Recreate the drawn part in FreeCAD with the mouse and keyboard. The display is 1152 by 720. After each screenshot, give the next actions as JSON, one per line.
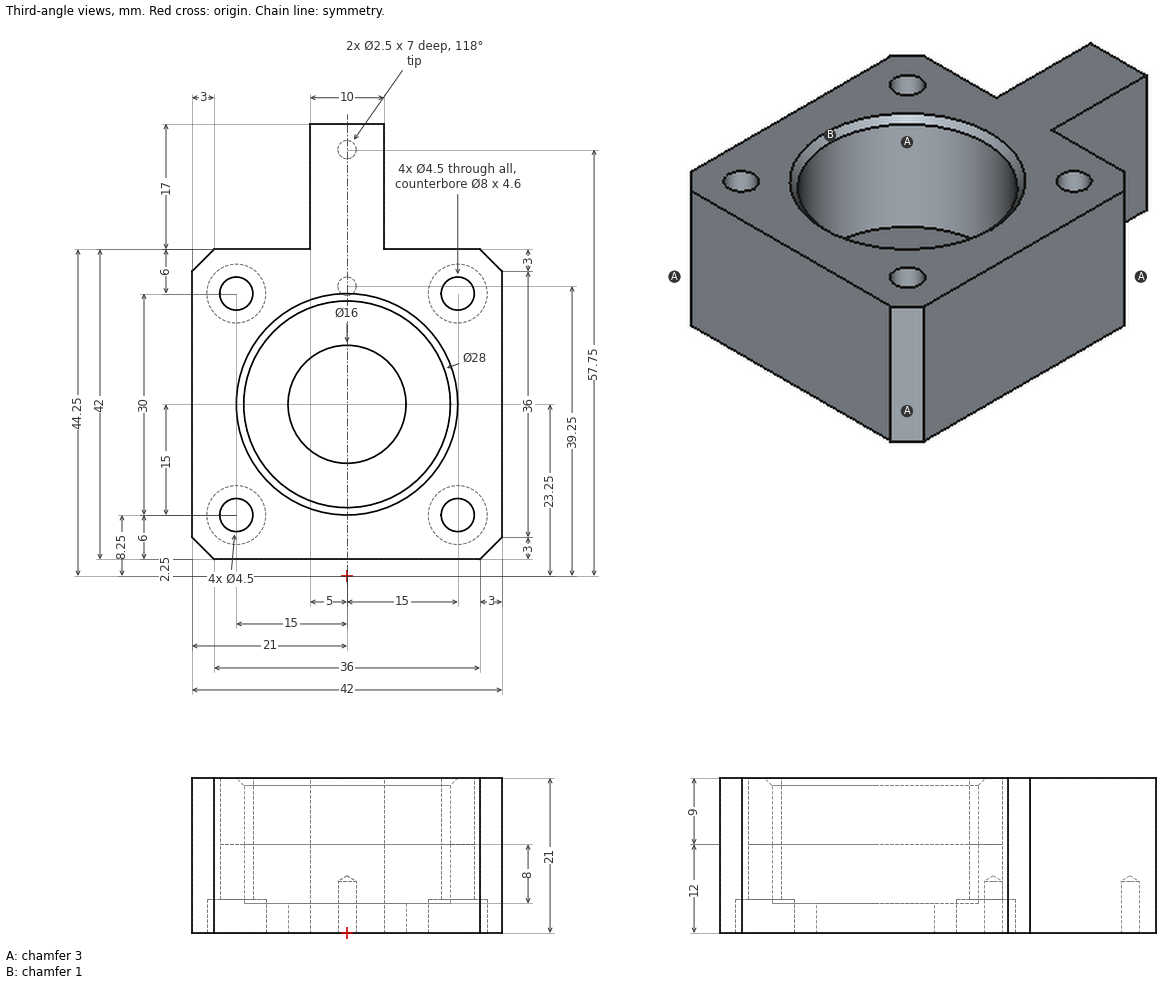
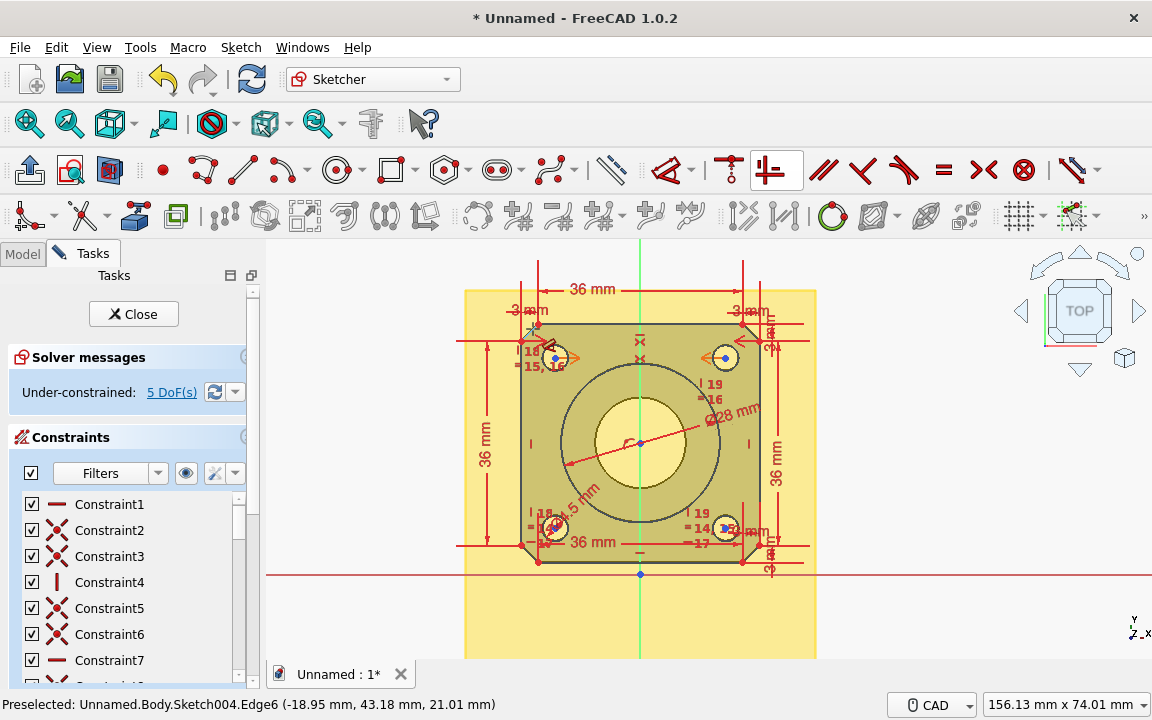
{"action": "left_click", "coordinate": [555, 529]}
{"action": "left_click", "coordinate": [598, 609]}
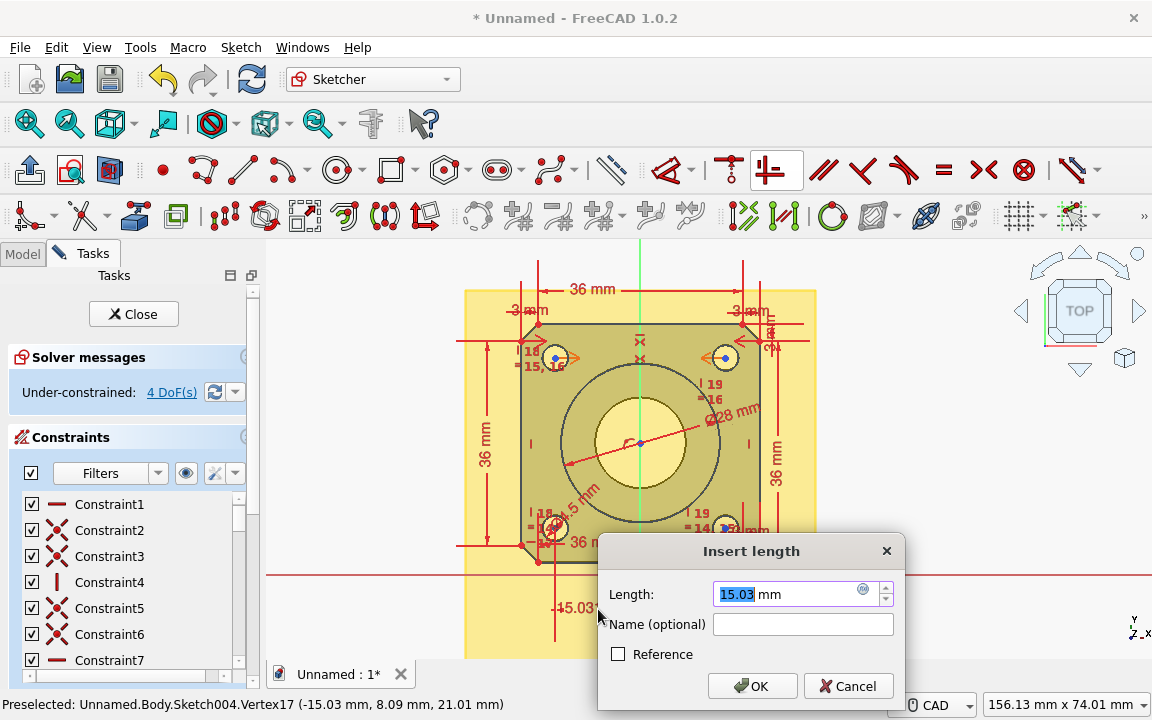
{"action": "type", "text": "15"}
{"action": "key", "text": "Return"}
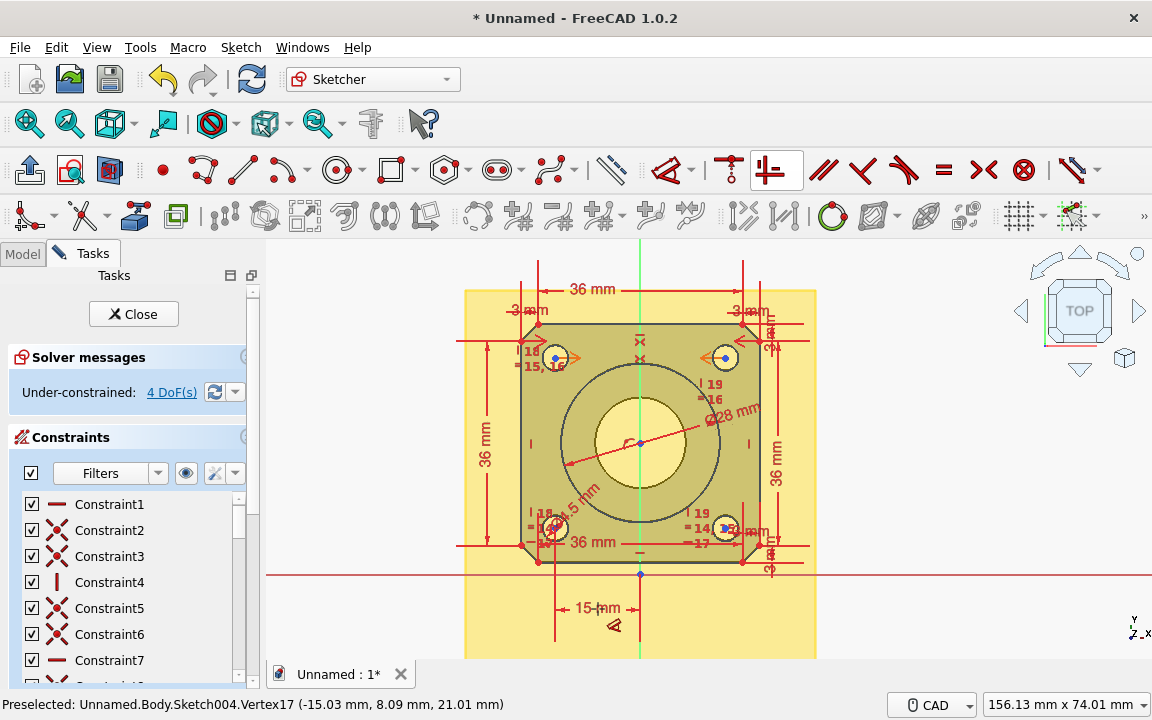
{"action": "left_click", "coordinate": [538, 563]}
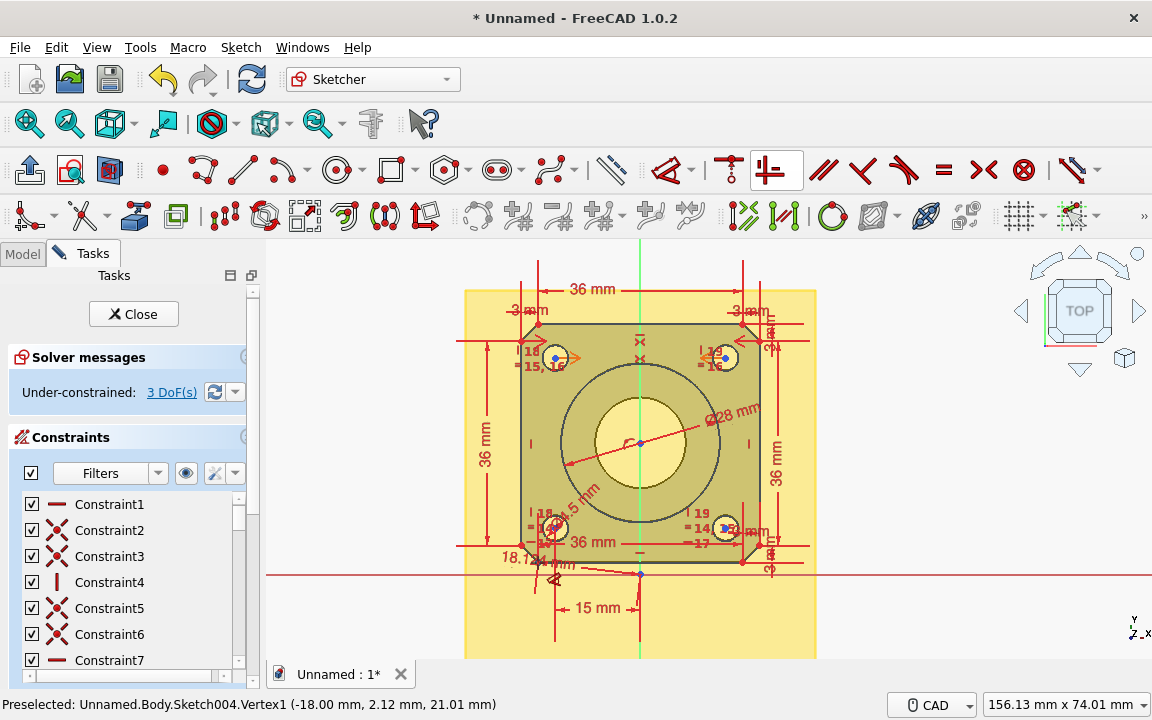
{"action": "left_click", "coordinate": [555, 529]}
{"action": "left_click", "coordinate": [504, 546]}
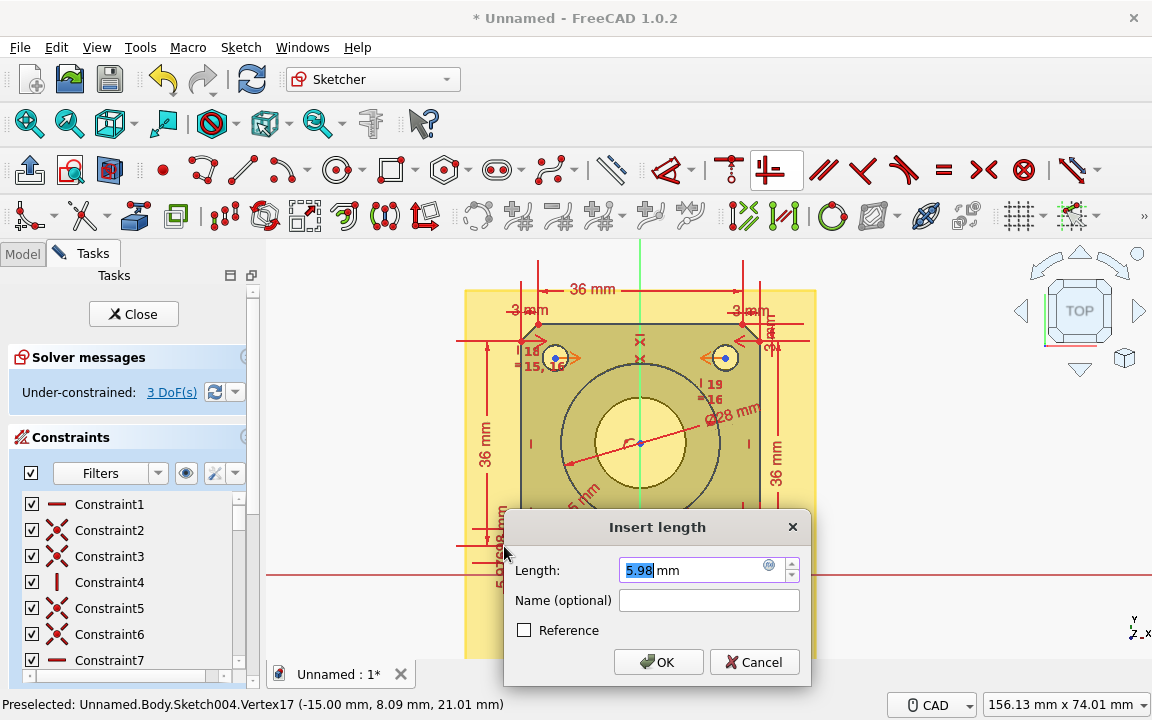
{"action": "type", "text": "6"}
{"action": "key", "text": "Return"}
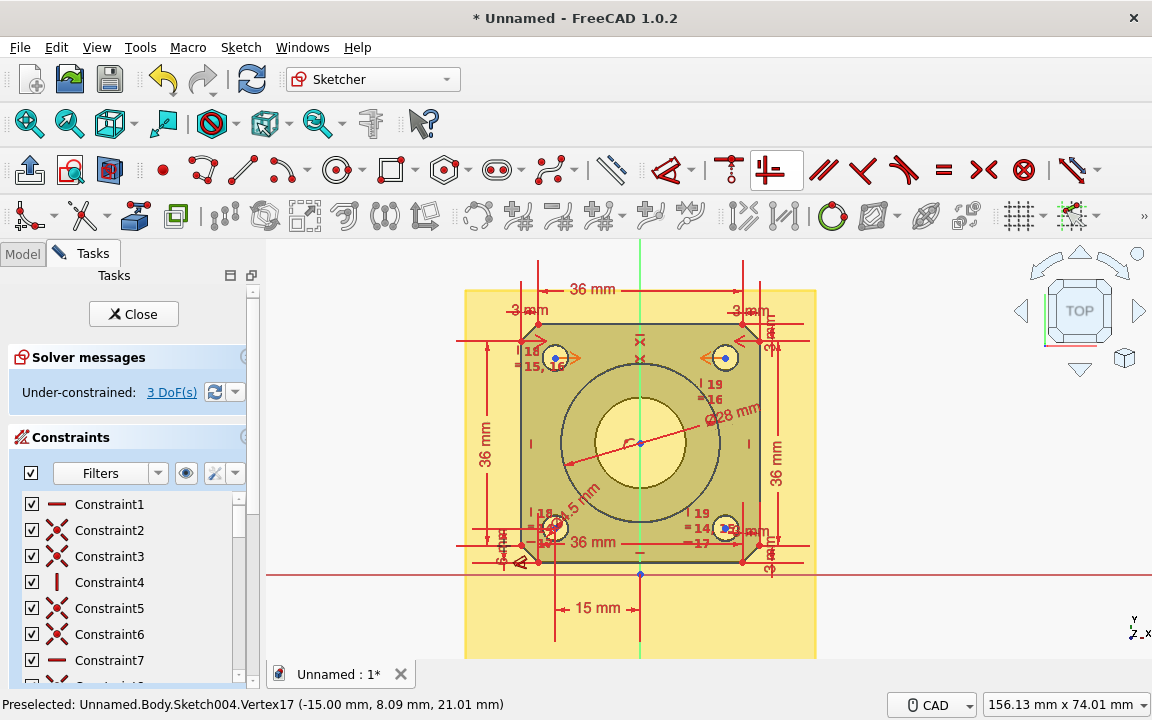
{"action": "left_click", "coordinate": [538, 324]}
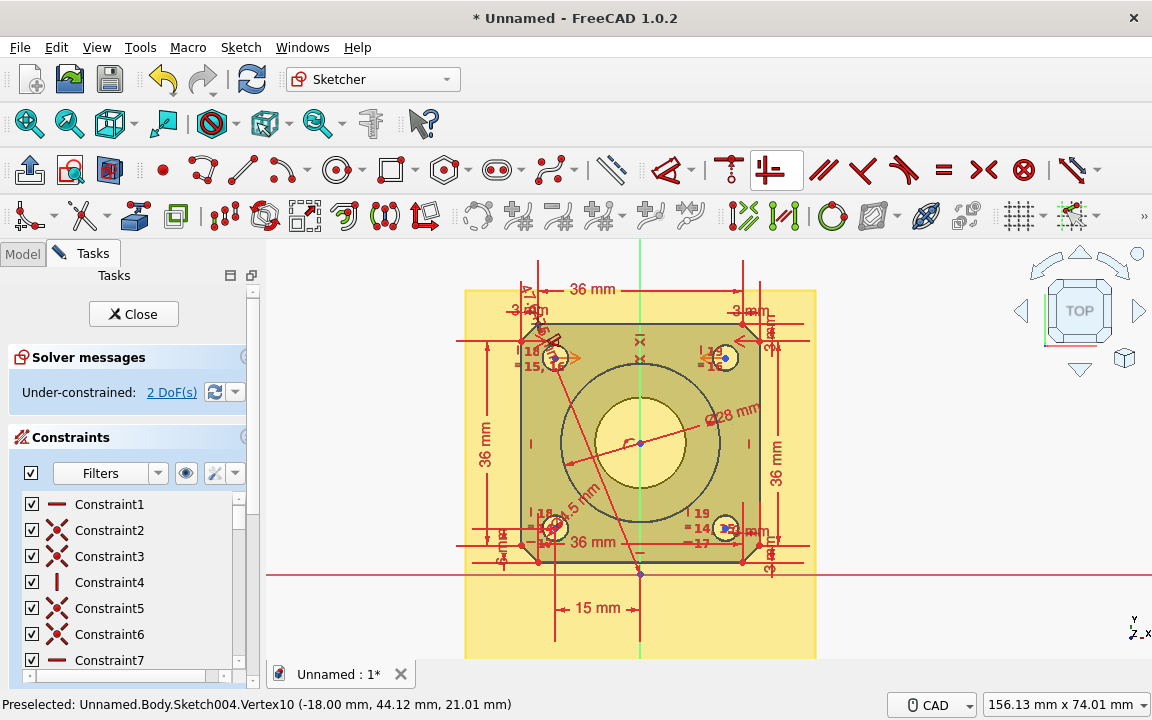
{"action": "left_click", "coordinate": [555, 358]}
{"action": "left_click", "coordinate": [504, 341]}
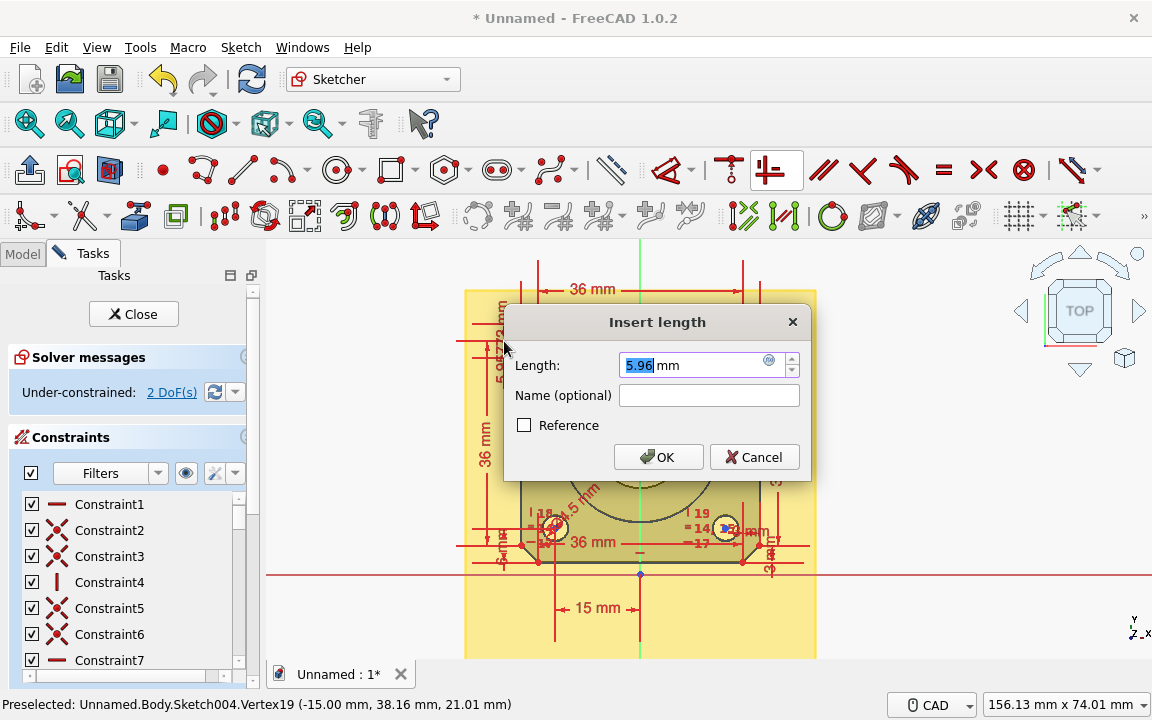
{"action": "type", "text": "6"}
{"action": "key", "text": "Return"}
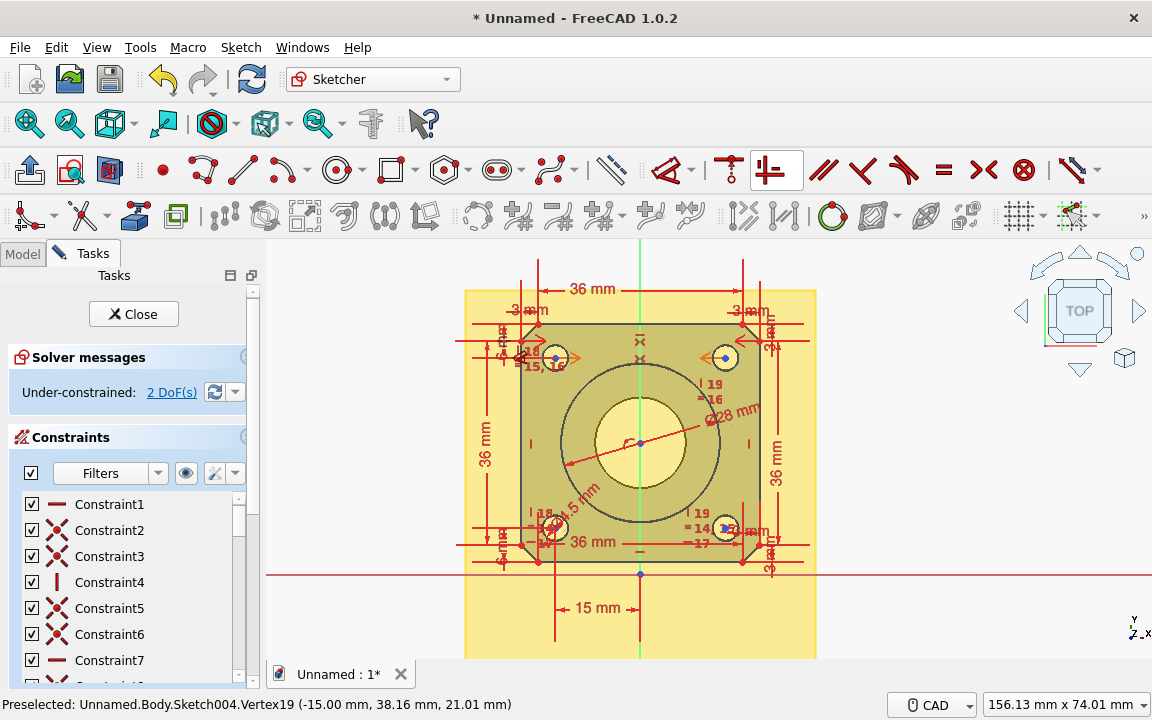
{"action": "left_click", "coordinate": [555, 528]}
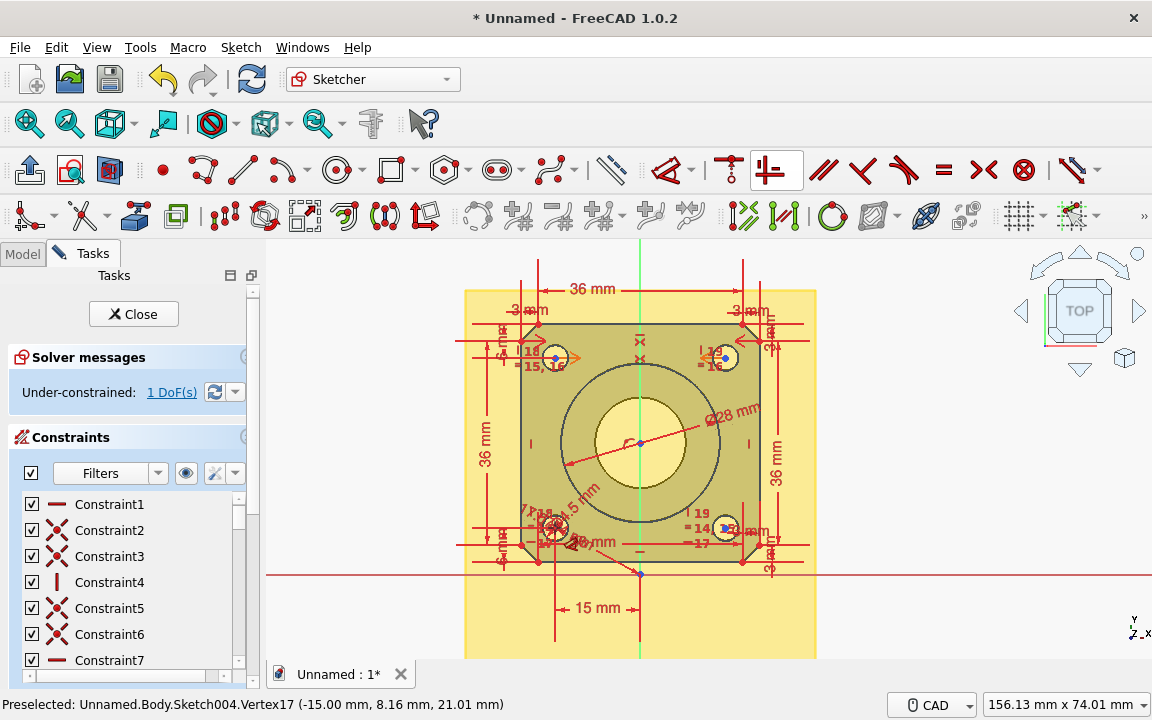
{"action": "left_click", "coordinate": [640, 443]}
{"action": "left_click", "coordinate": [674, 486]}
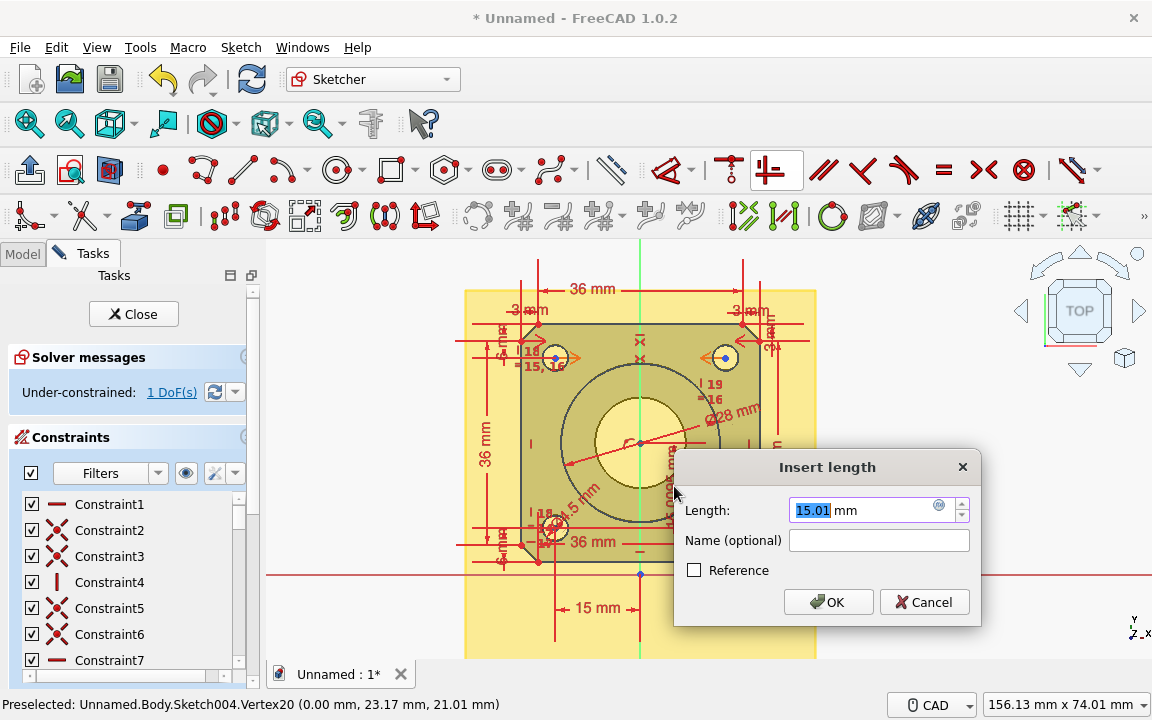
{"action": "type", "text": "15"}
{"action": "key", "text": "Return"}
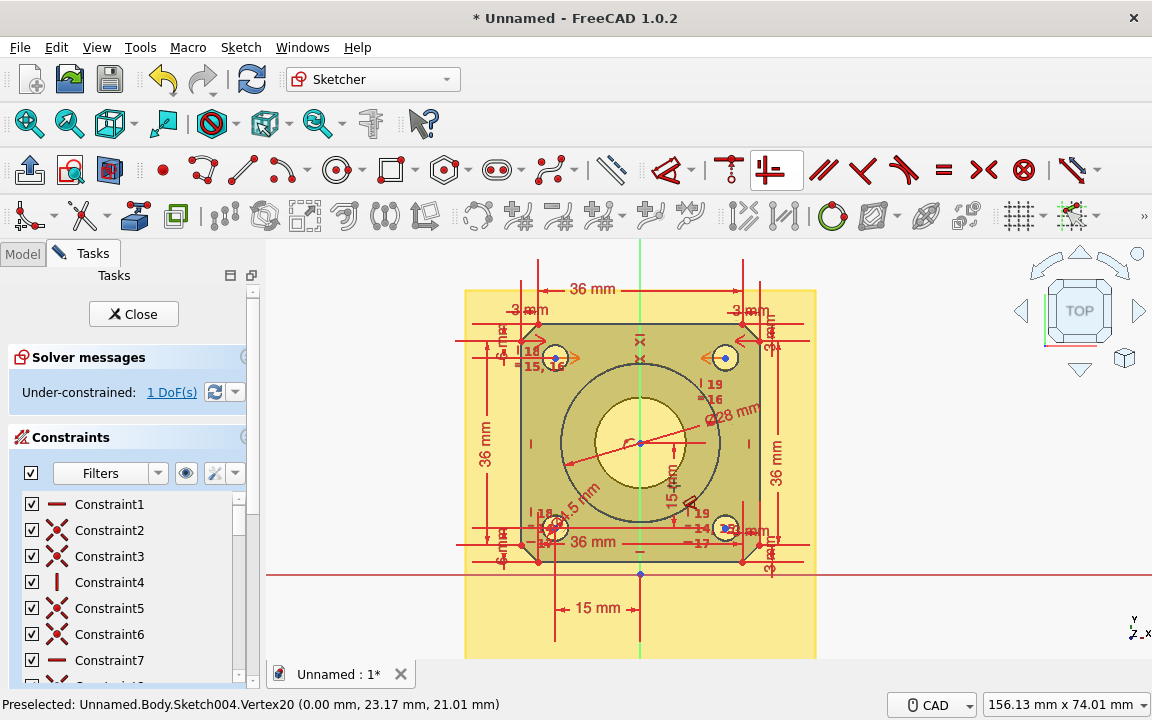
{"action": "left_click", "coordinate": [555, 528]}
{"action": "left_click", "coordinate": [674, 541]}